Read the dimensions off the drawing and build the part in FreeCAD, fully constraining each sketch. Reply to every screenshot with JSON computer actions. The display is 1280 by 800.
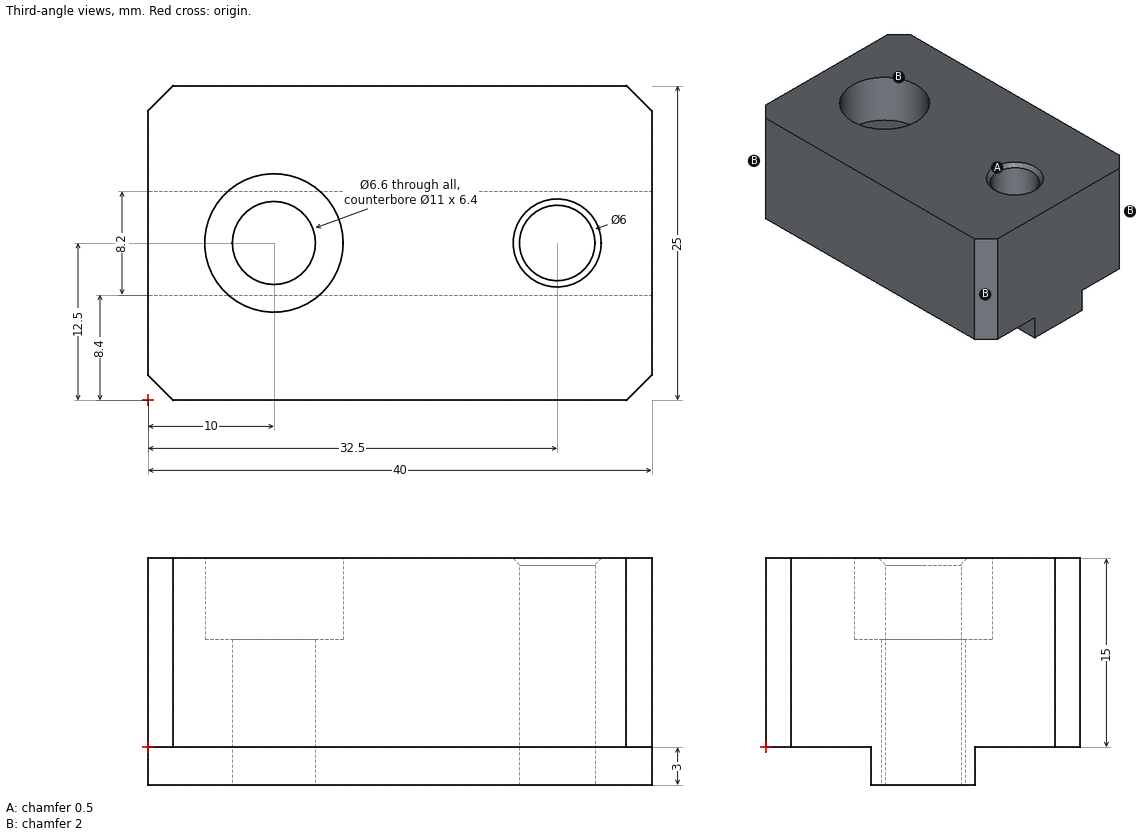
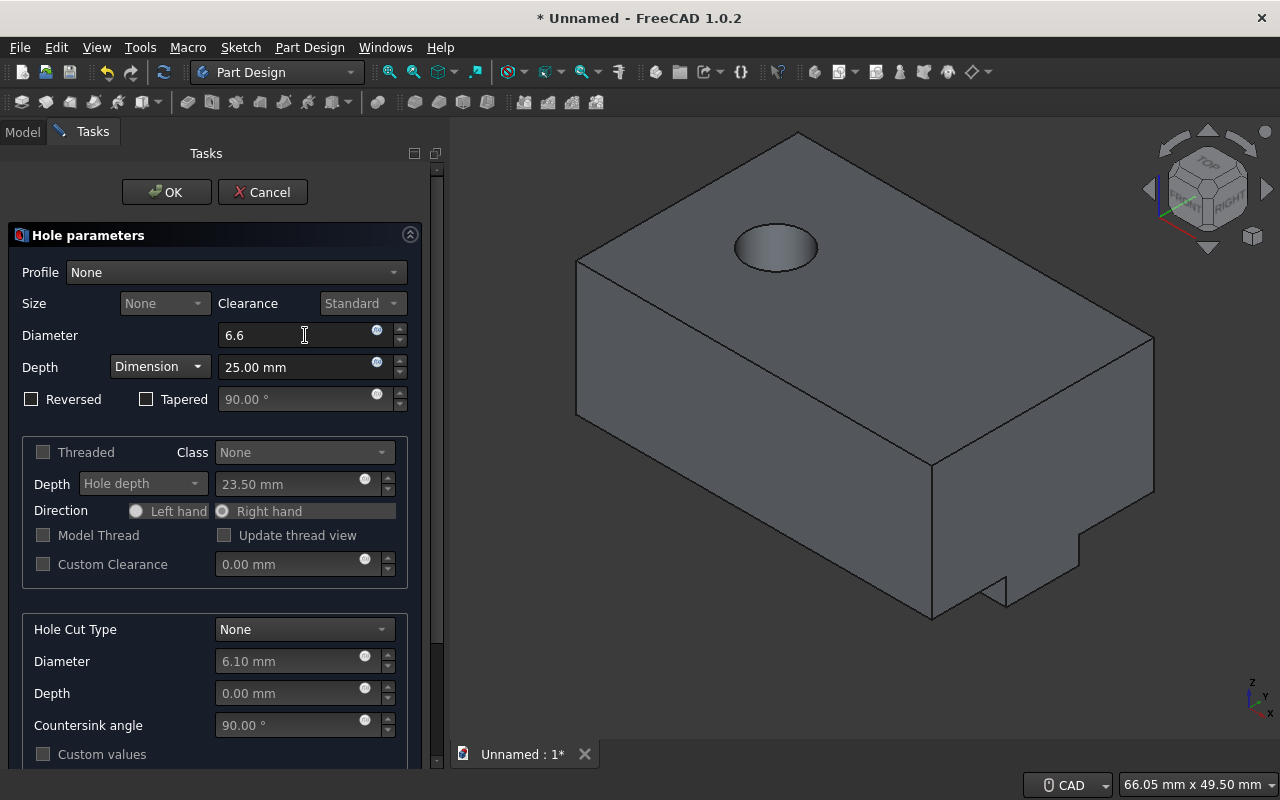
{"action": "left_click", "coordinate": [161, 366]}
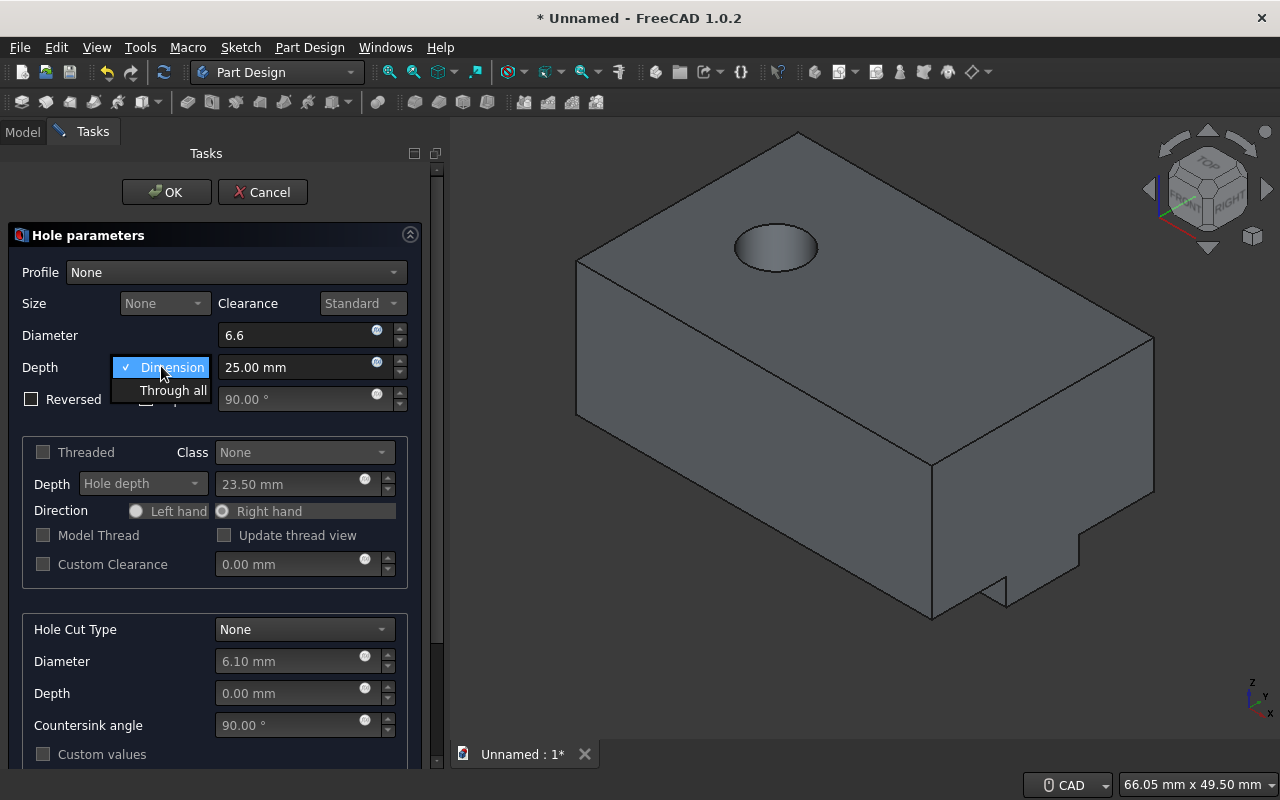
{"action": "left_click", "coordinate": [160, 390]}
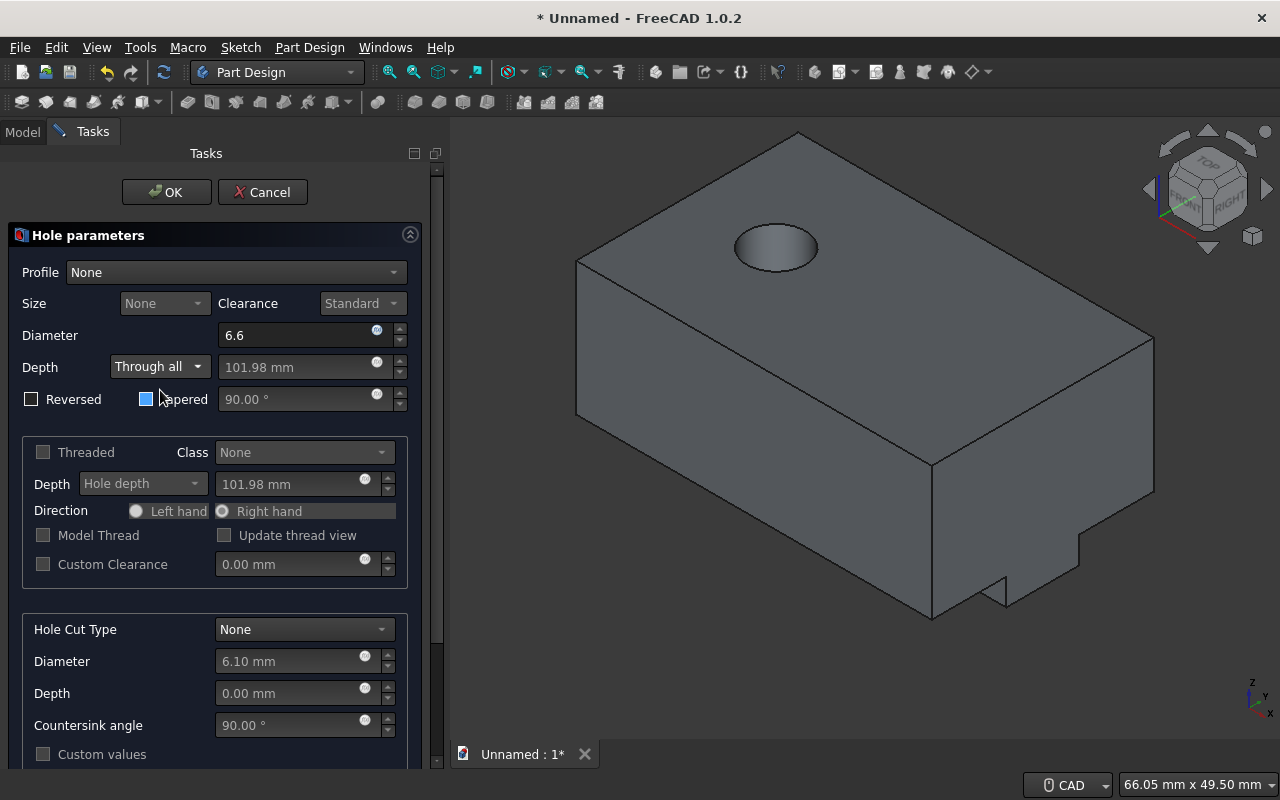
{"action": "left_click", "coordinate": [306, 630]}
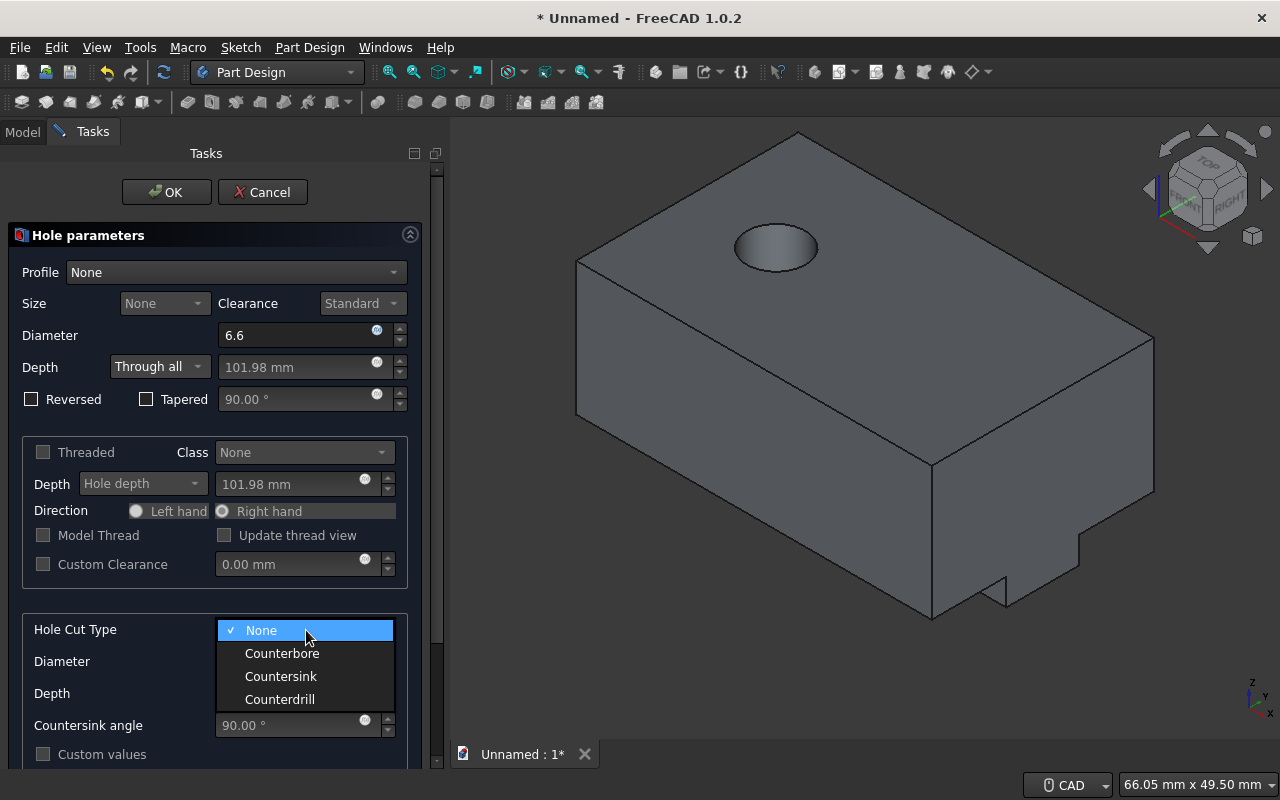
{"action": "left_click", "coordinate": [304, 654]}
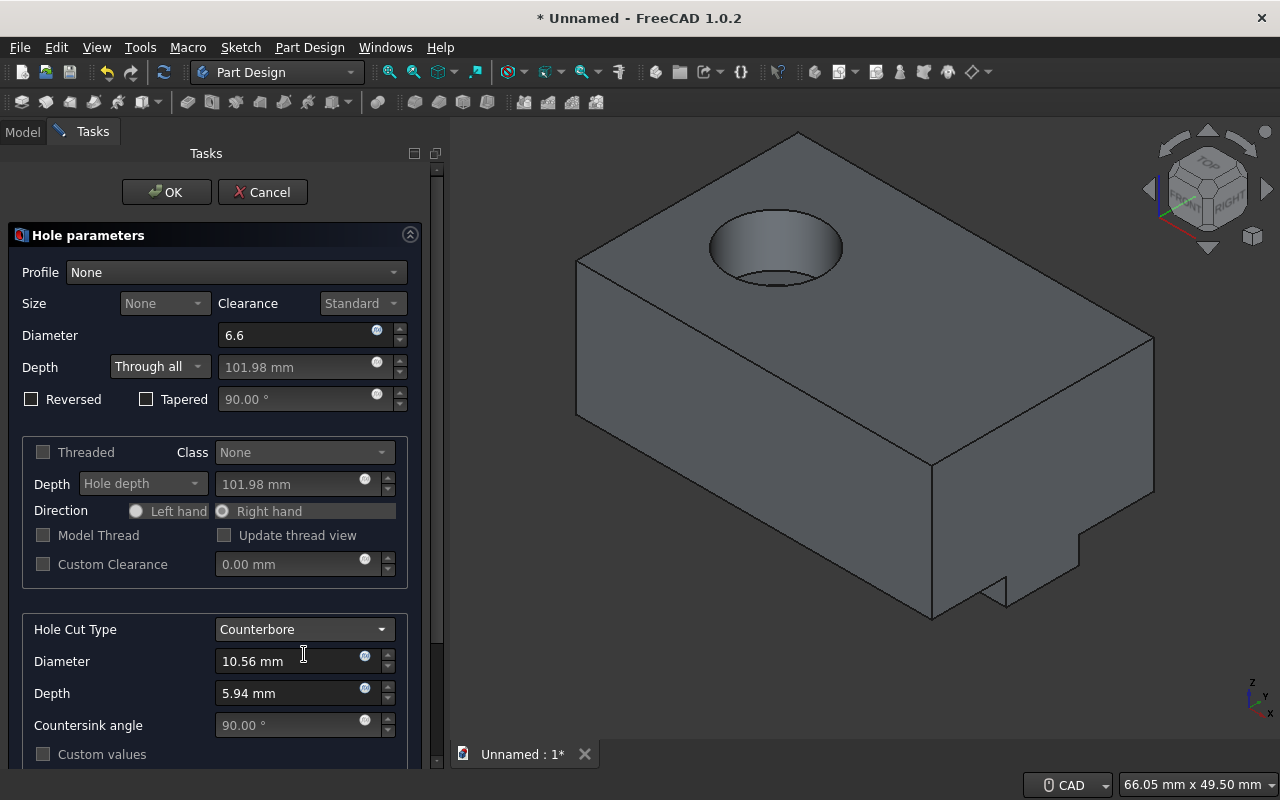
{"action": "triple_click", "coordinate": [298, 661]}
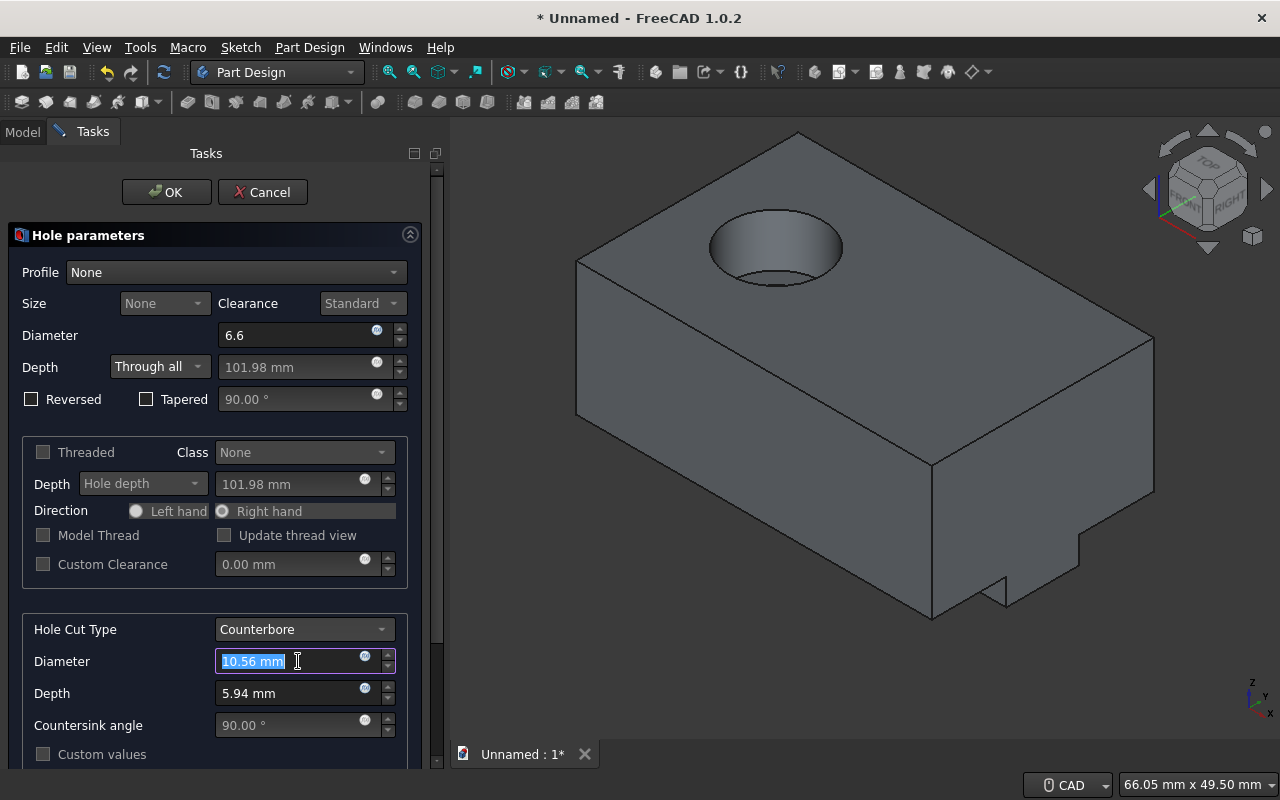
{"action": "type", "text": "11"}
{"action": "key", "text": "Tab"}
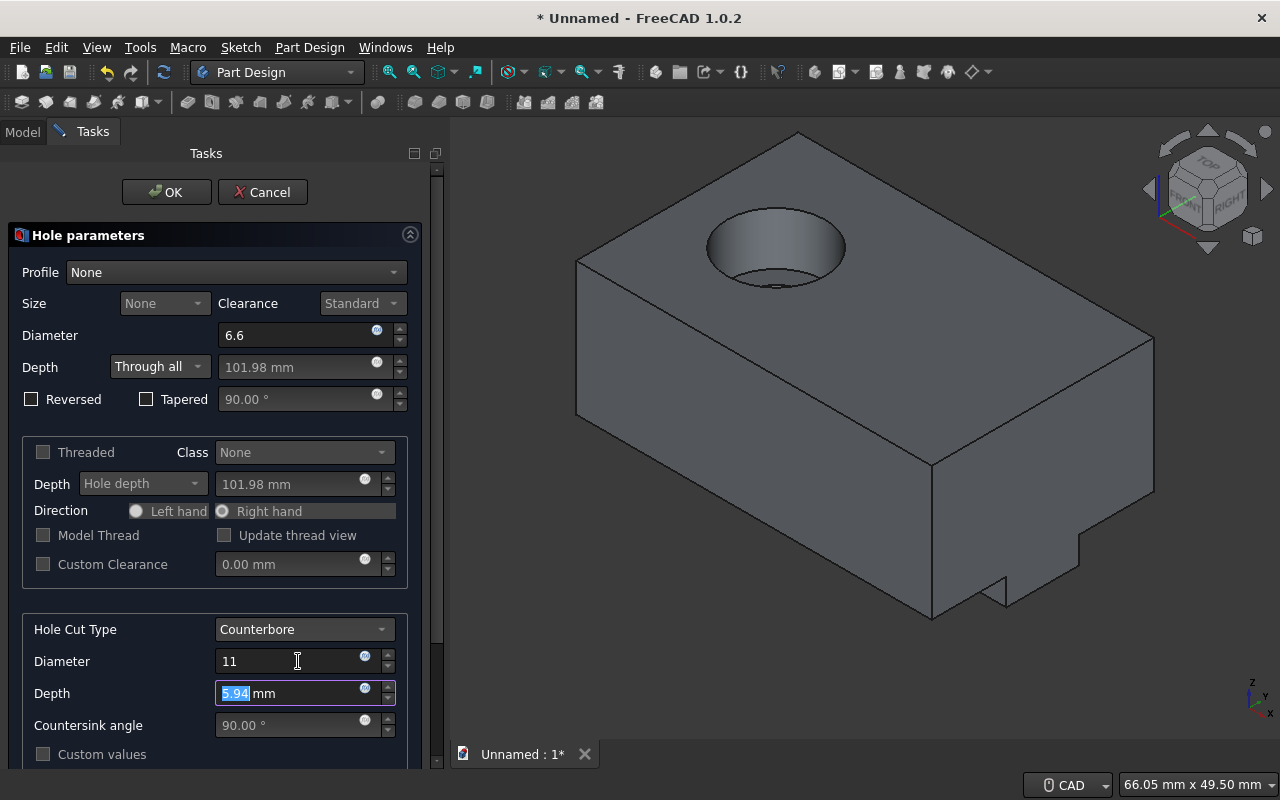
{"action": "type", "text": "6.4"}
{"action": "key", "text": "Tab"}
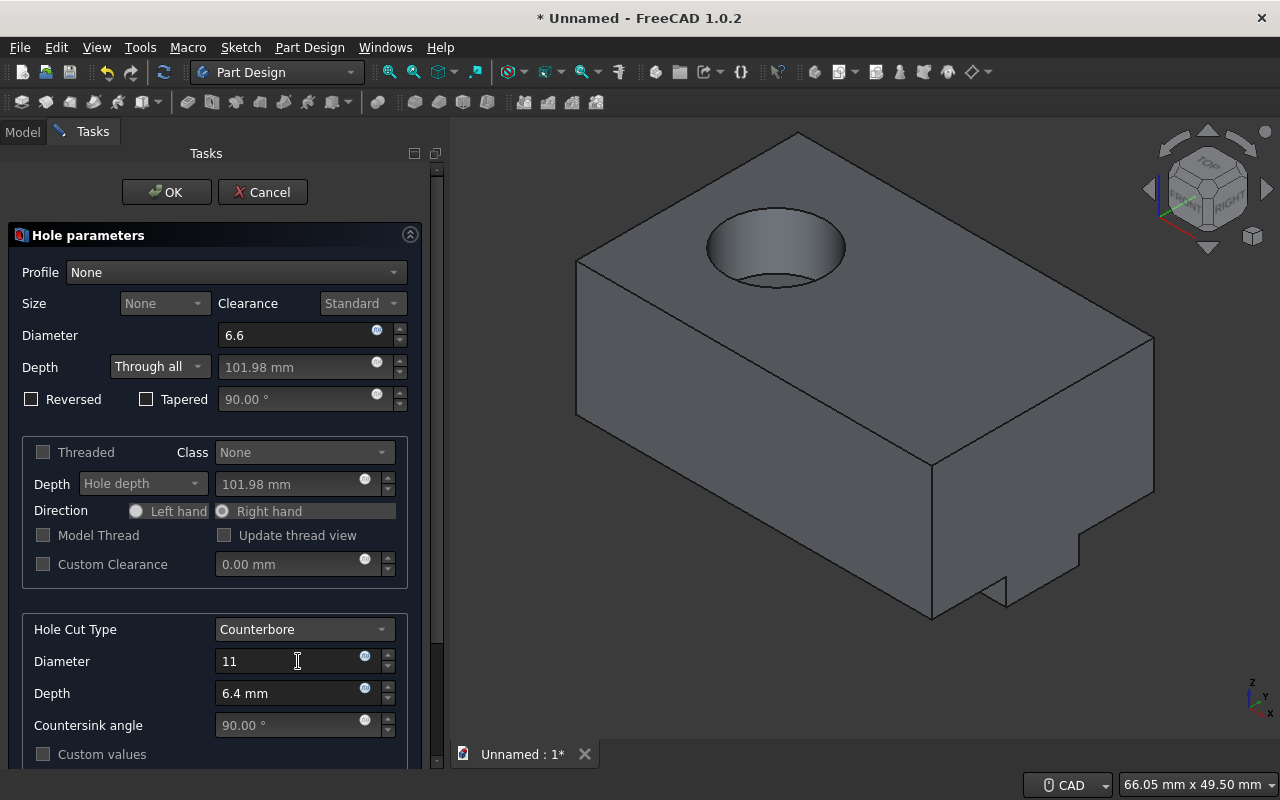
{"action": "left_click", "coordinate": [167, 192]}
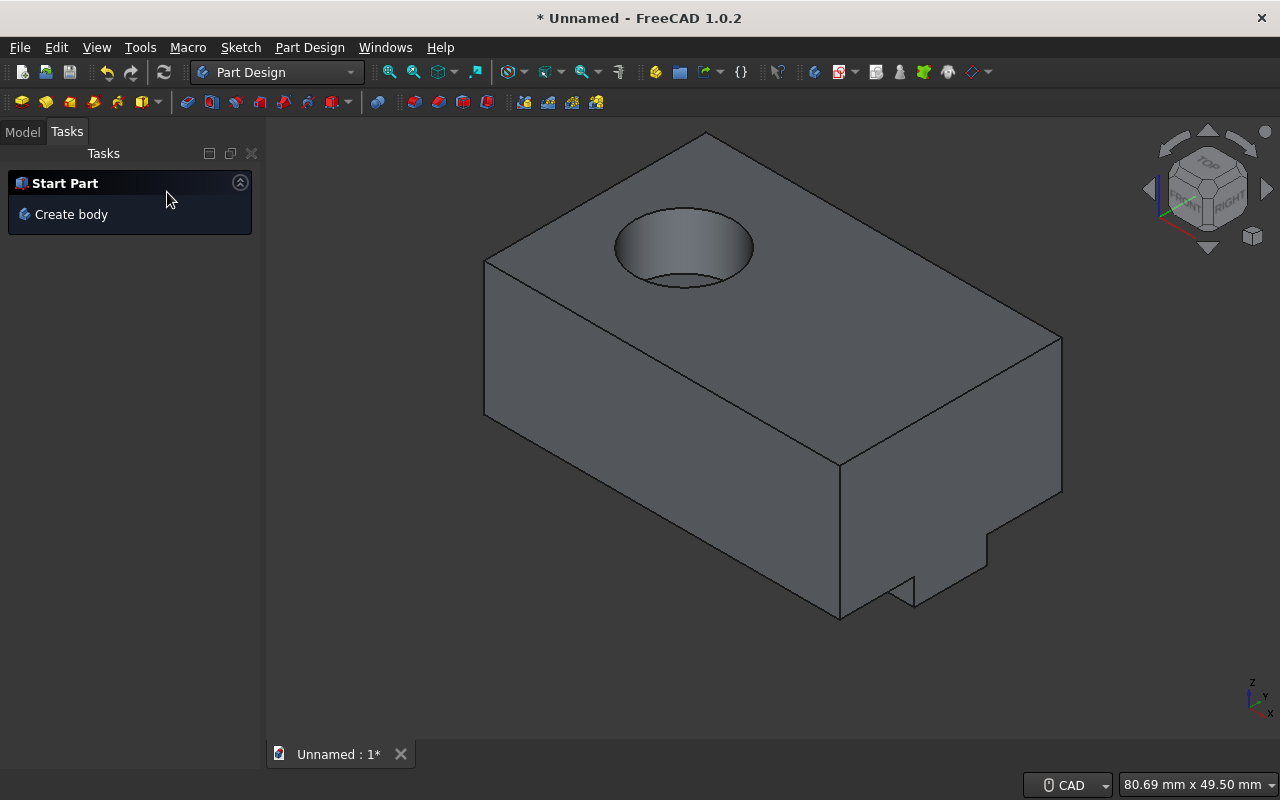
{"action": "left_click", "coordinate": [824, 327]}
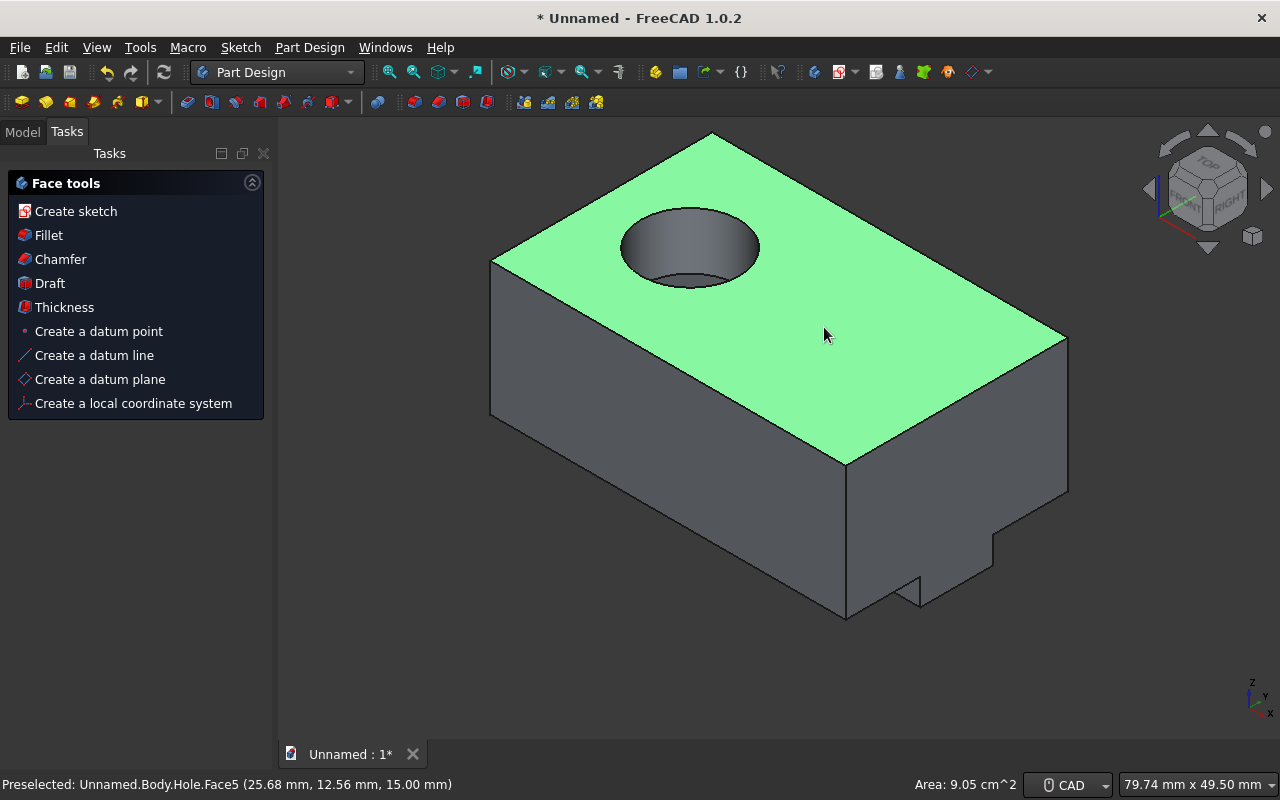
{"action": "left_click", "coordinate": [840, 72]}